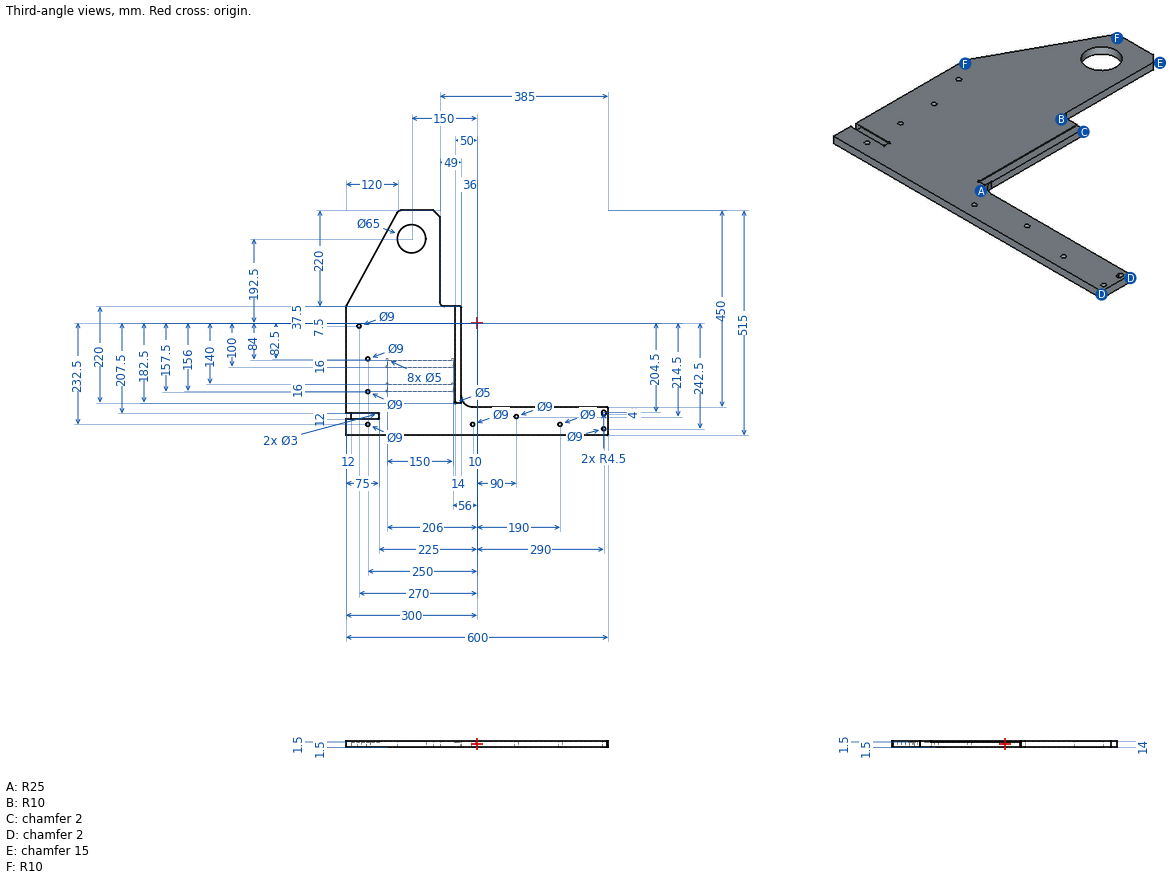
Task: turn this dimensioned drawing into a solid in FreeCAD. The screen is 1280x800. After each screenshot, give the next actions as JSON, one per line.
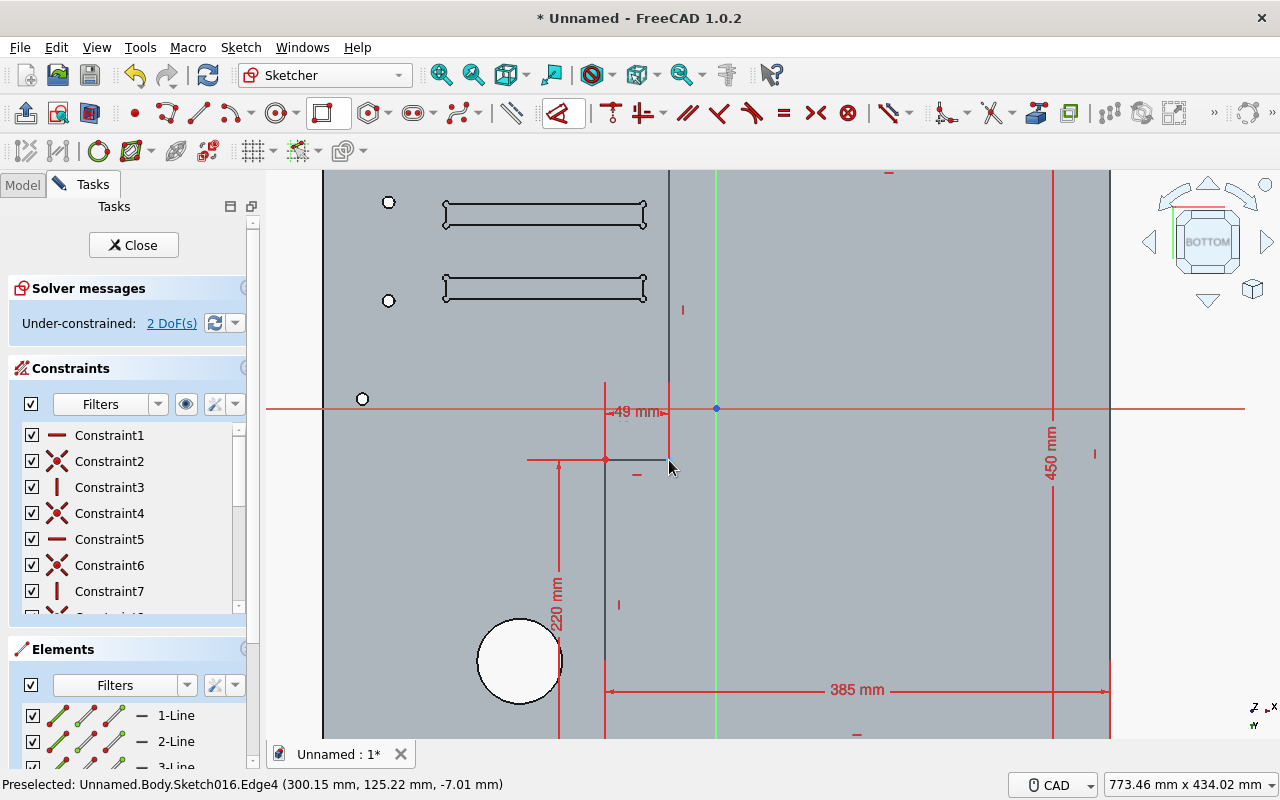
{"action": "left_click", "coordinate": [669, 460]}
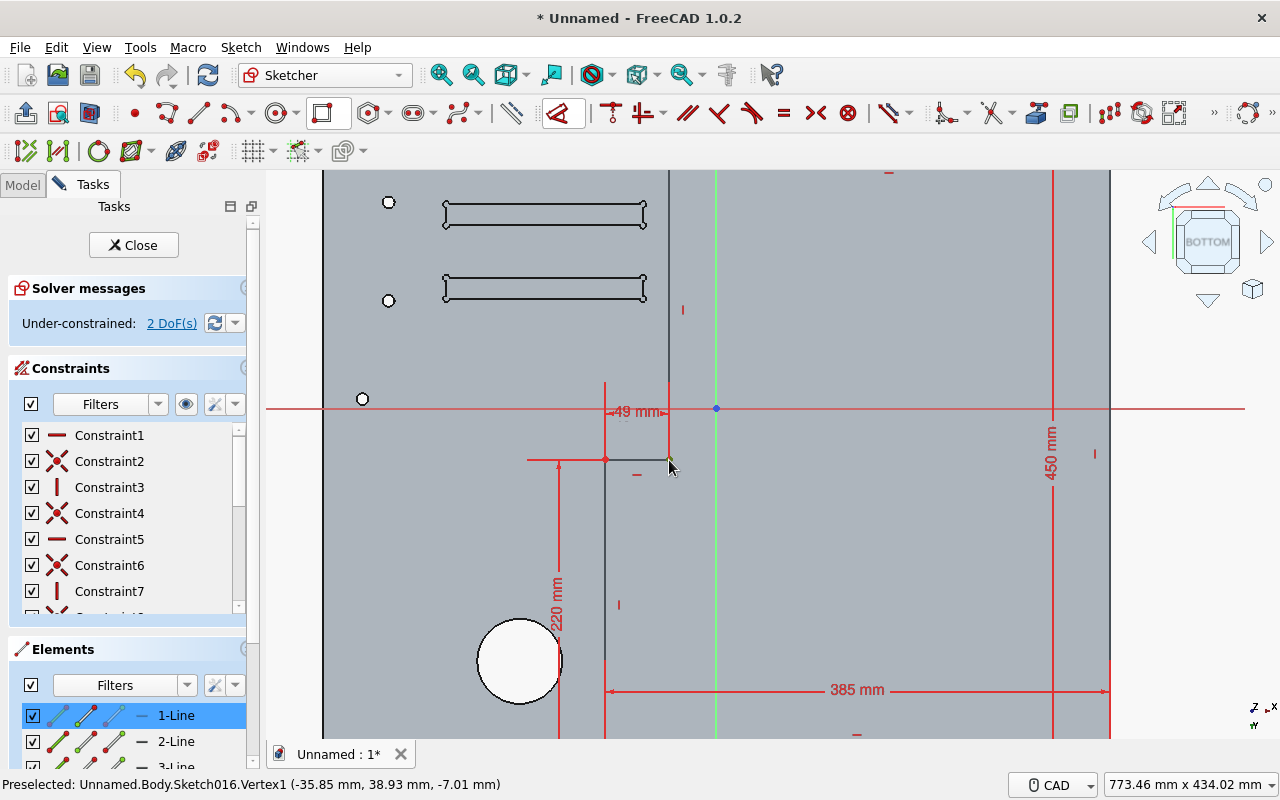
{"action": "key", "text": "l"}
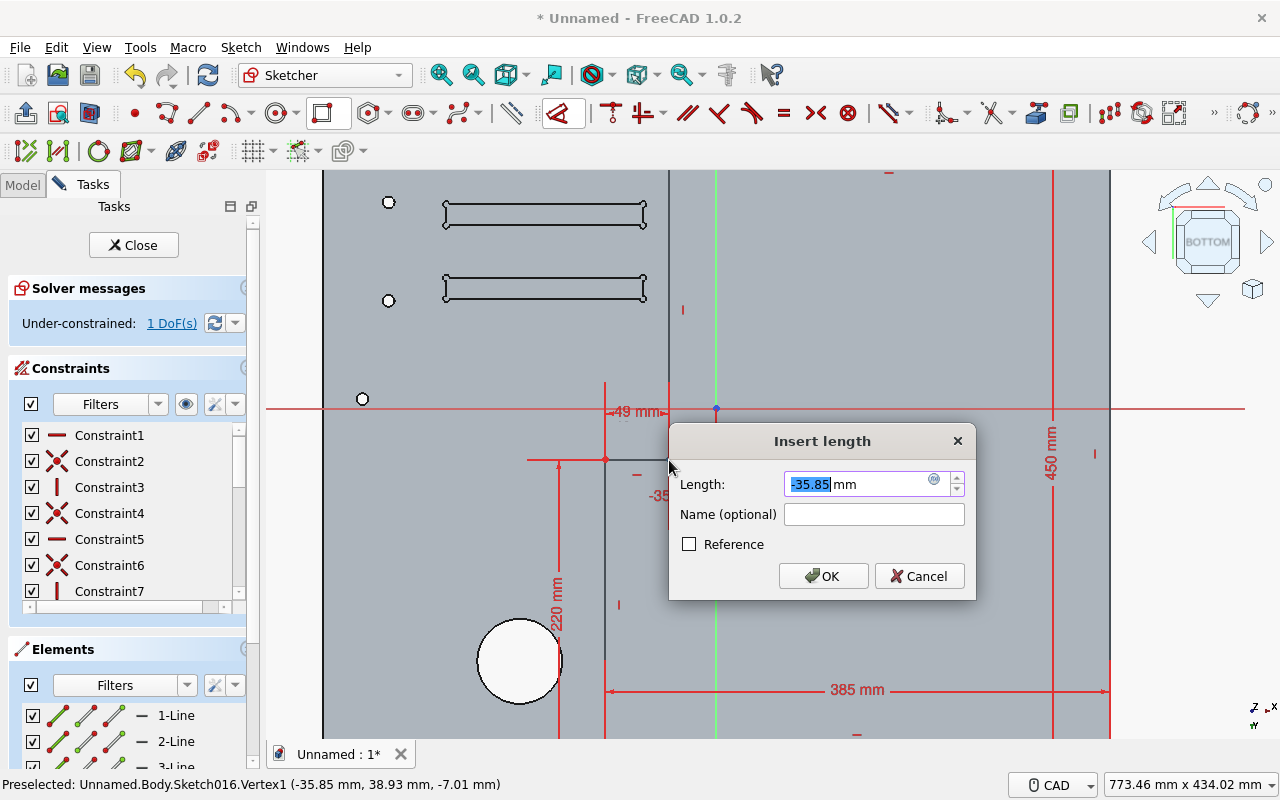
{"action": "type", "text": "-36"}
{"action": "key", "text": "Return"}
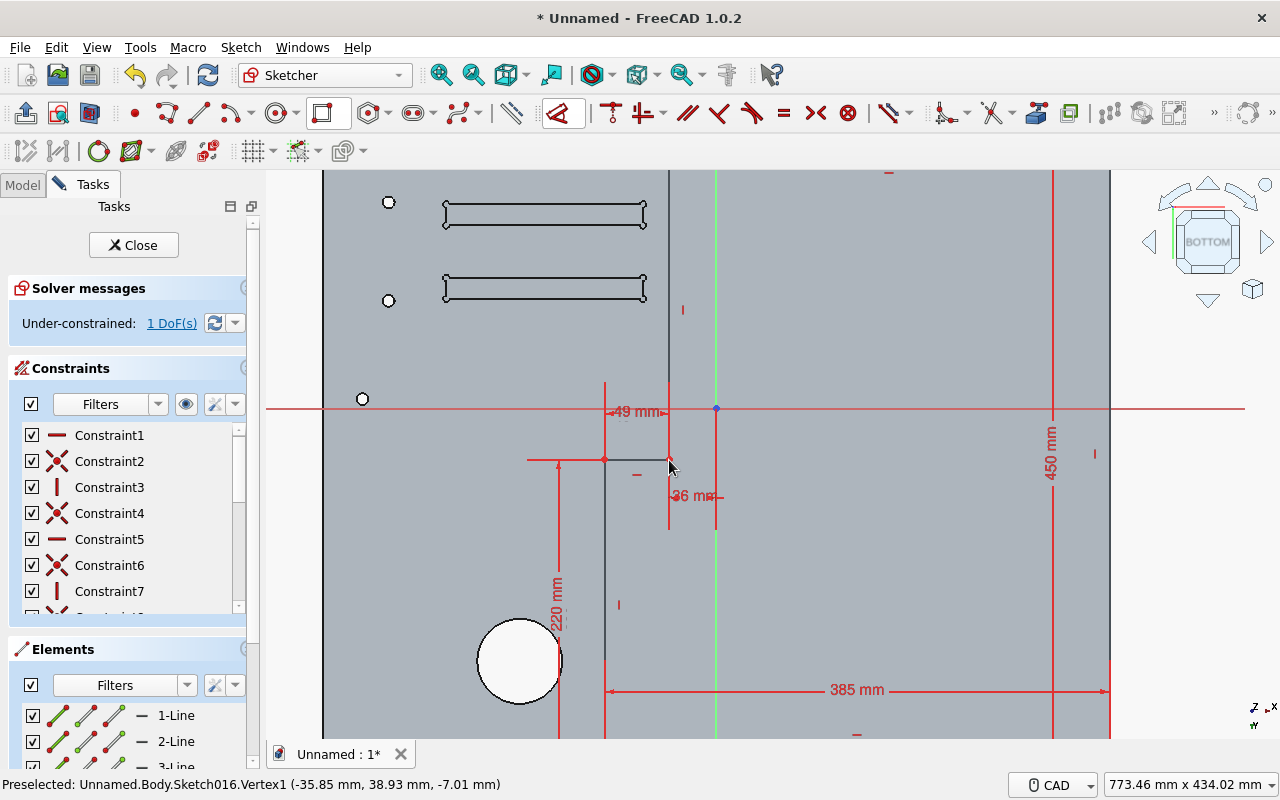
{"action": "left_click", "coordinate": [669, 460]}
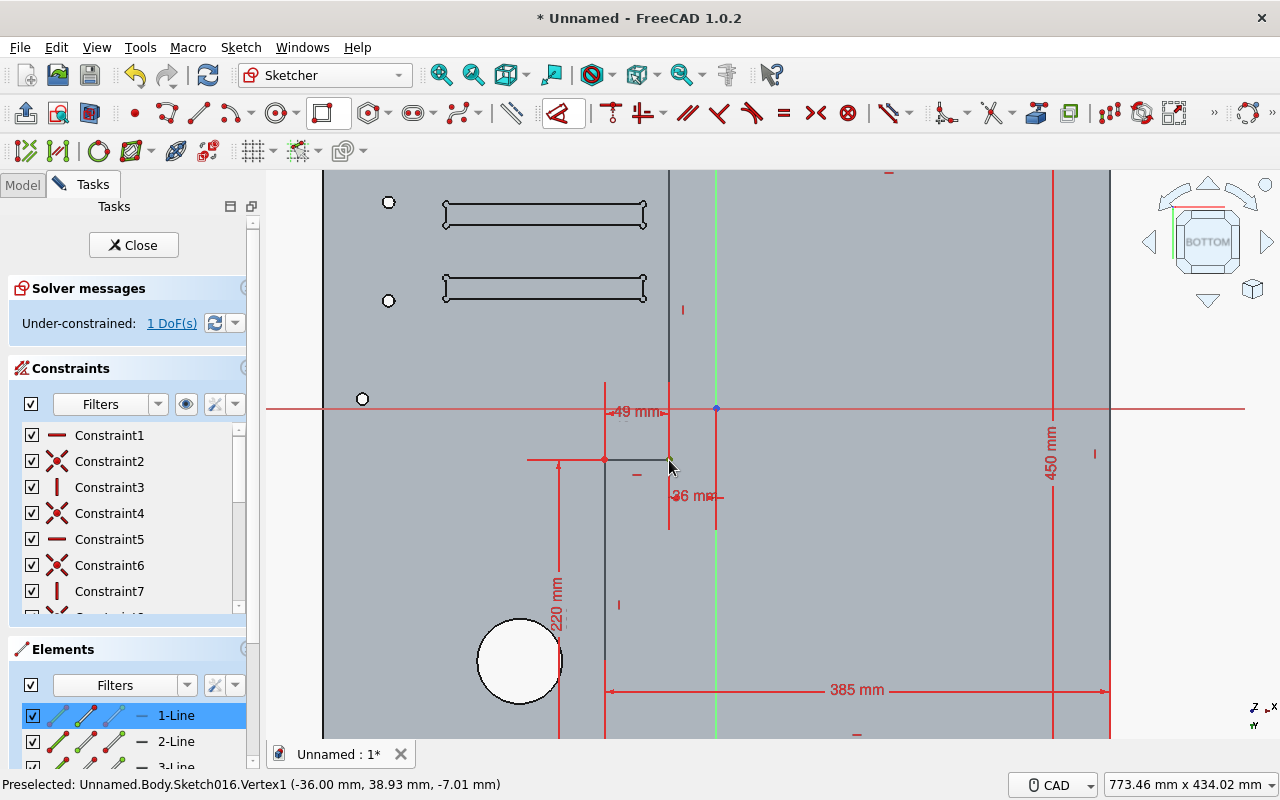
{"action": "left_click", "coordinate": [580, 114]}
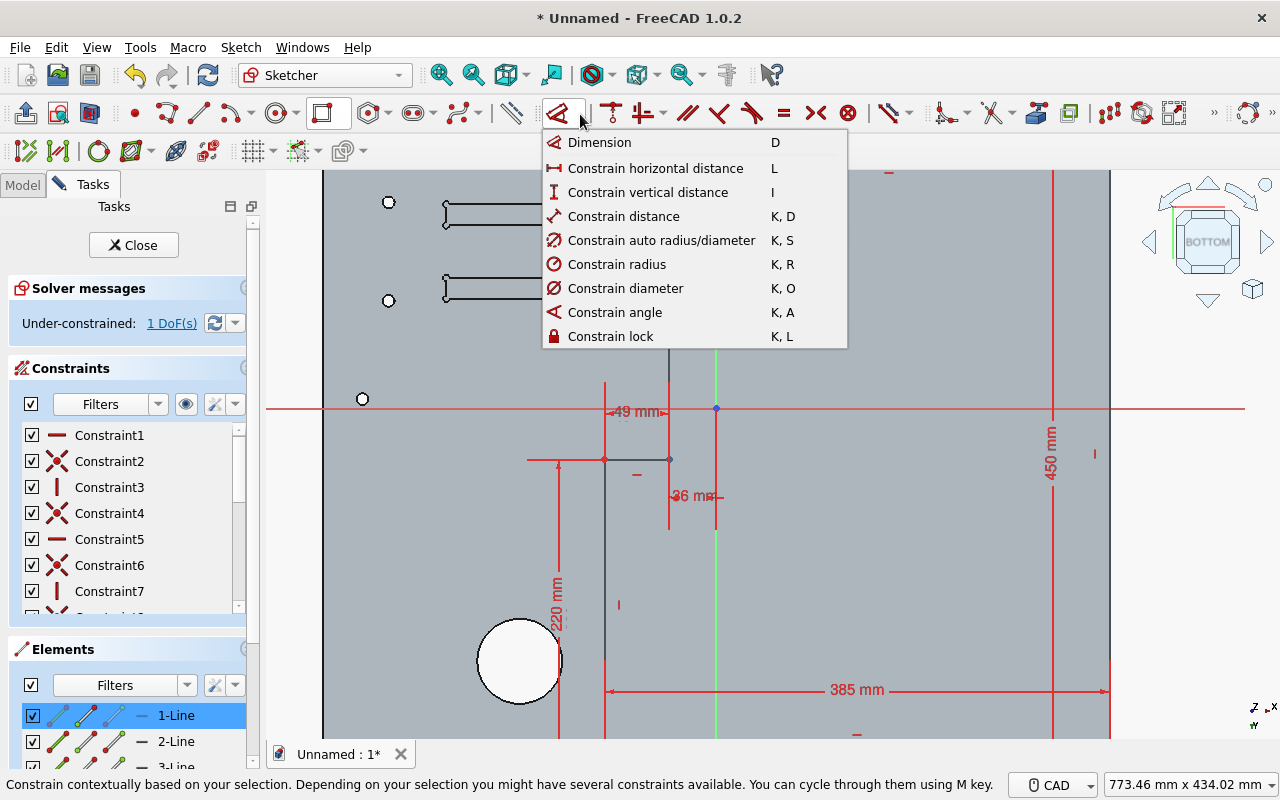
{"action": "left_click", "coordinate": [695, 192]}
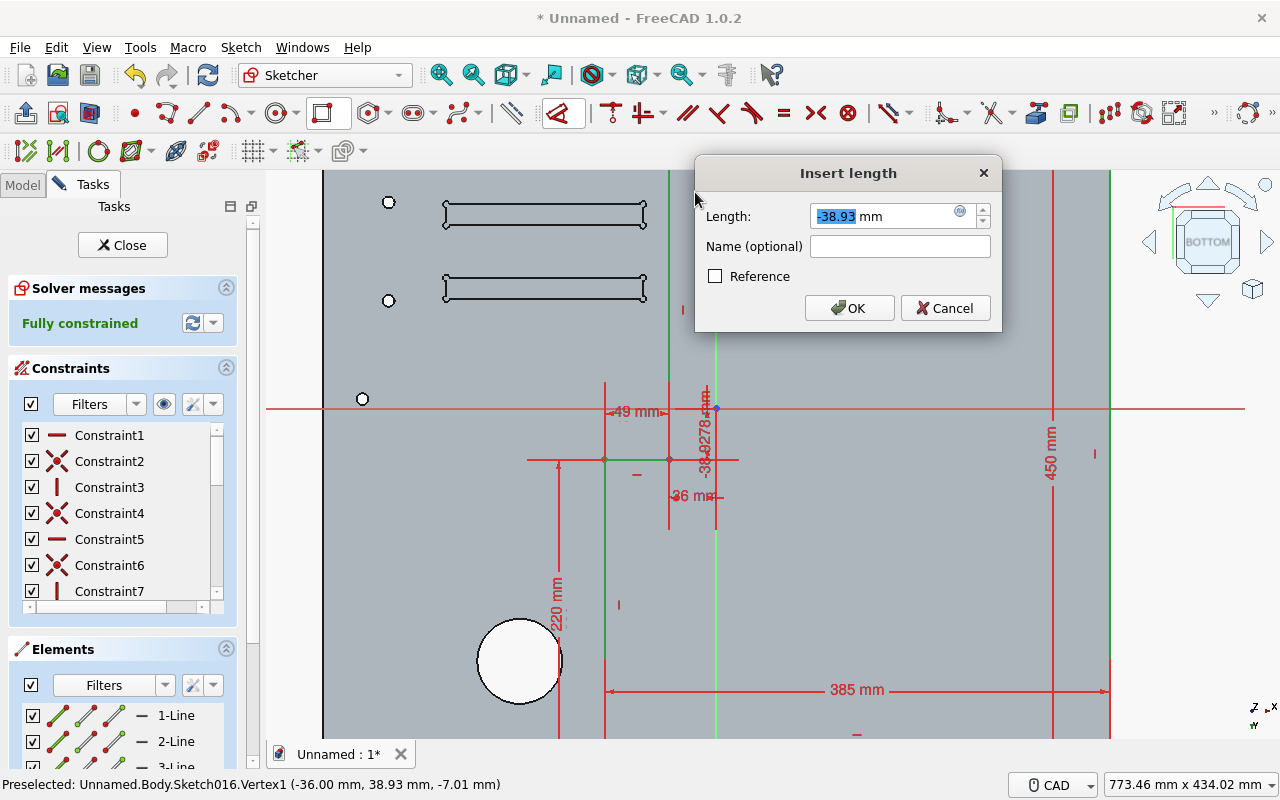
{"action": "type", "text": "-37.5"}
{"action": "key", "text": "Return"}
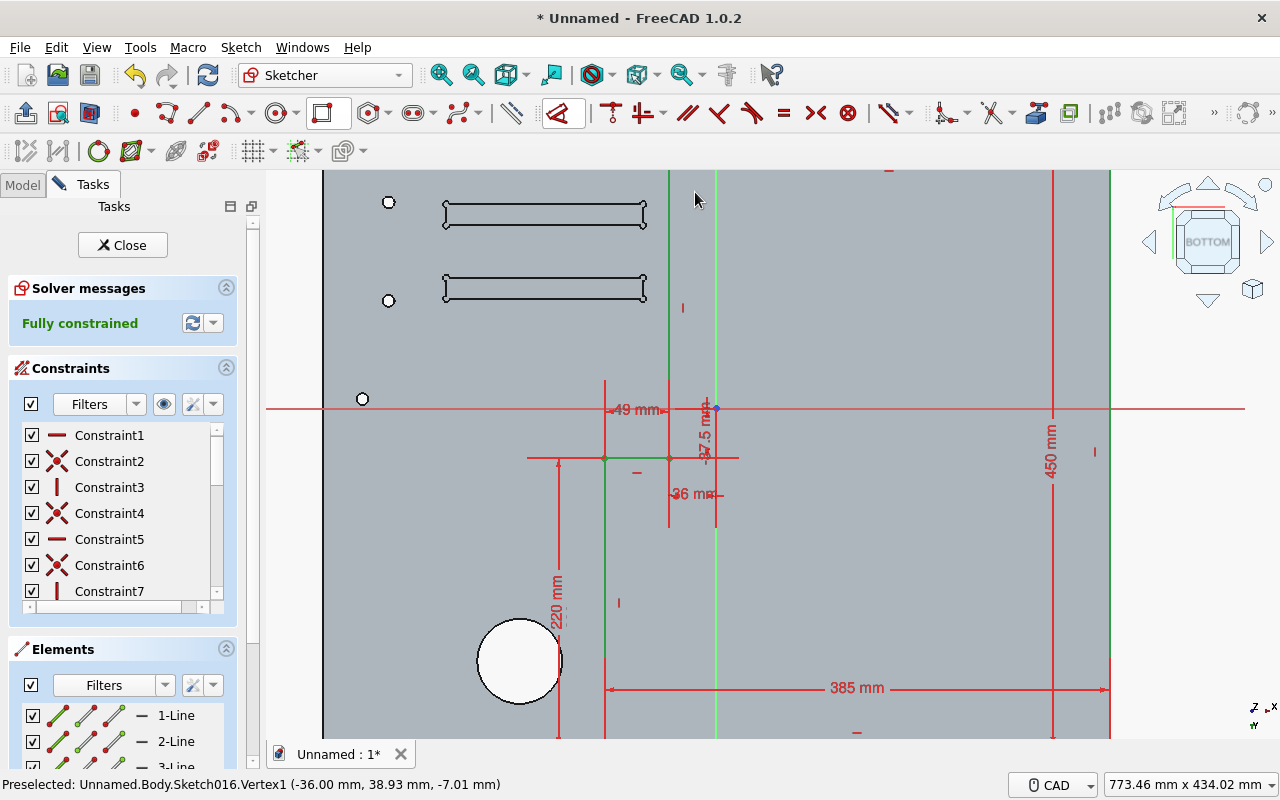
{"action": "left_click", "coordinate": [123, 245]}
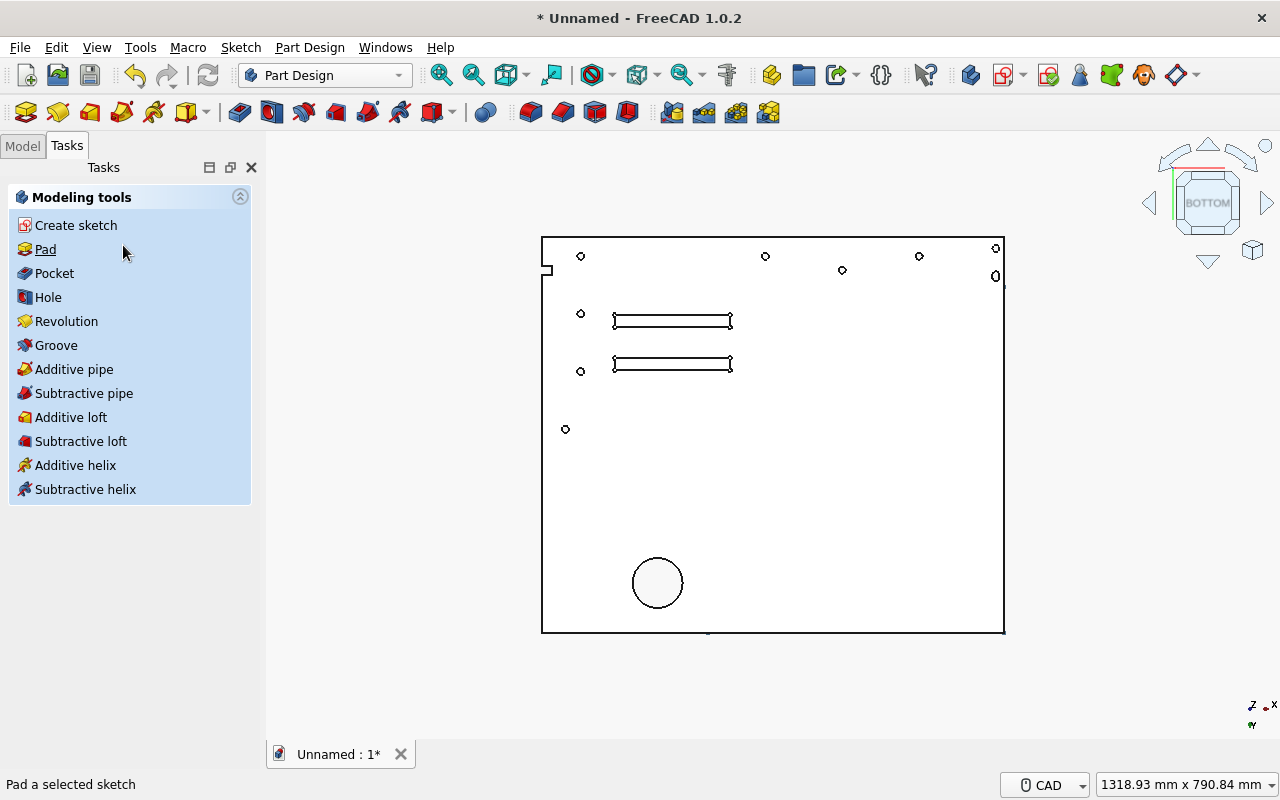
{"action": "left_click", "coordinate": [240, 112]}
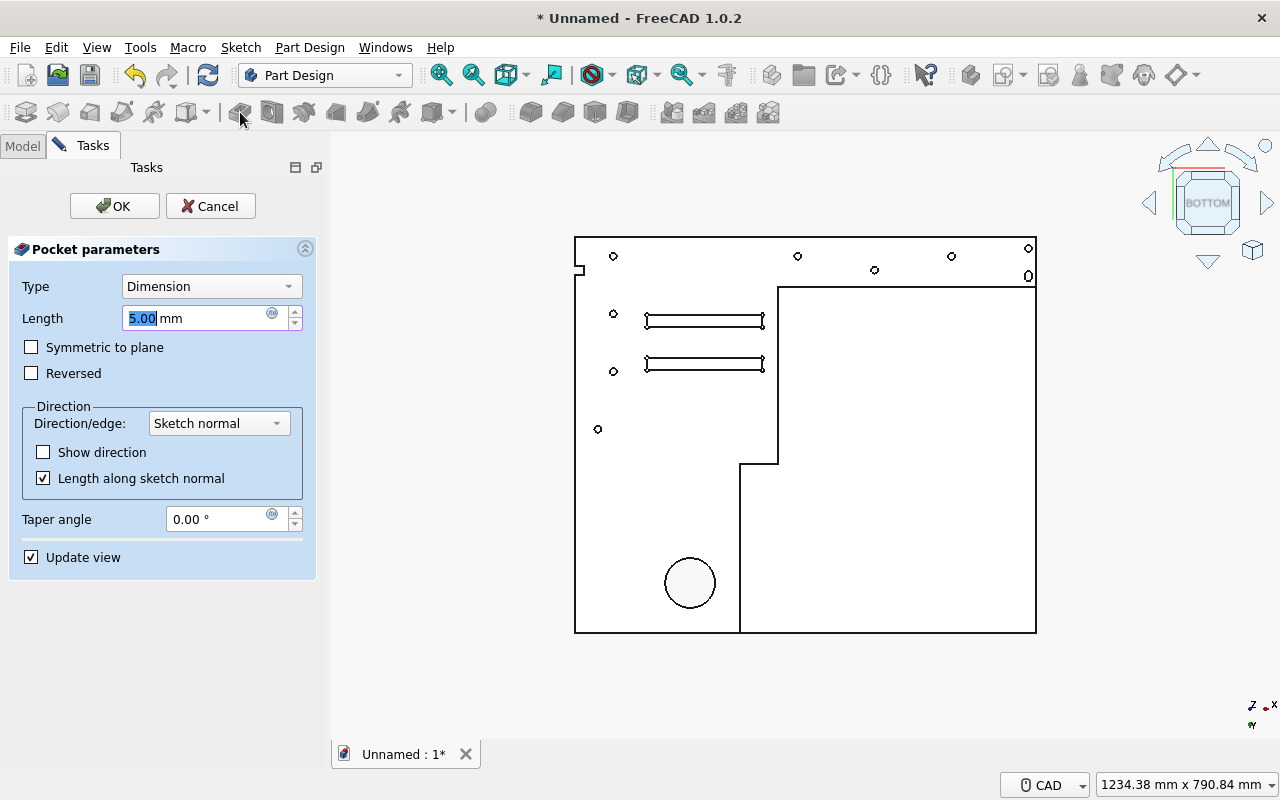
{"action": "left_click", "coordinate": [212, 286]}